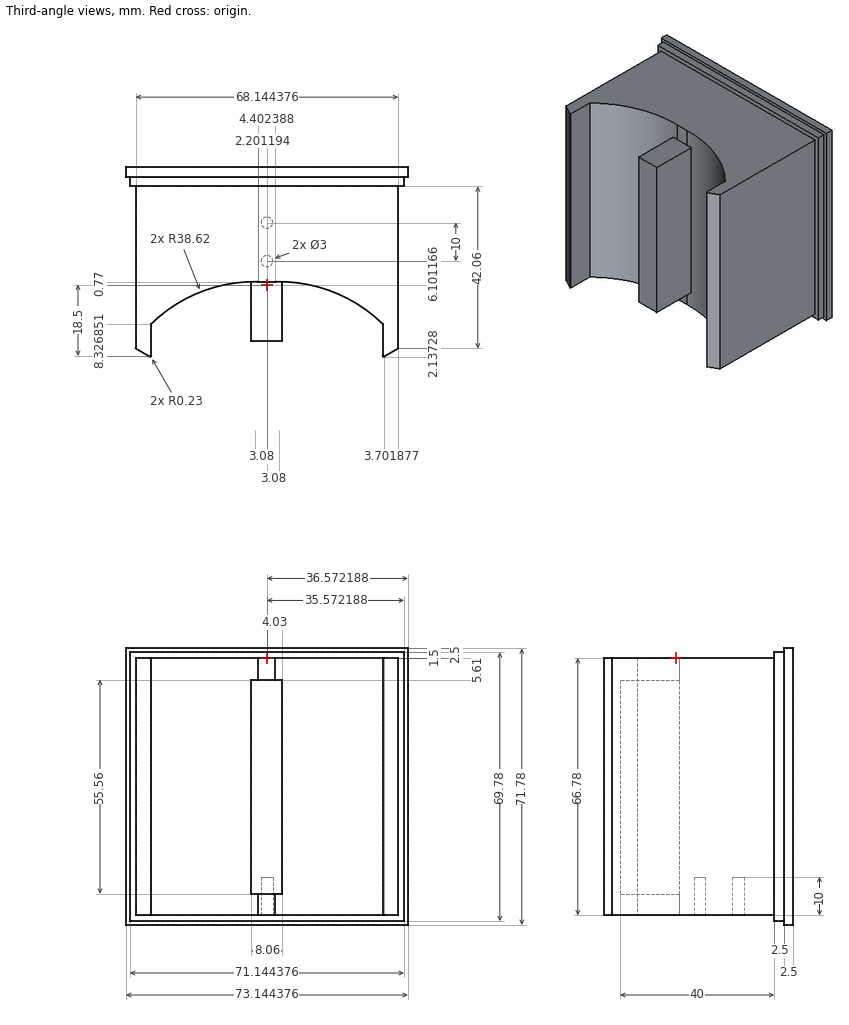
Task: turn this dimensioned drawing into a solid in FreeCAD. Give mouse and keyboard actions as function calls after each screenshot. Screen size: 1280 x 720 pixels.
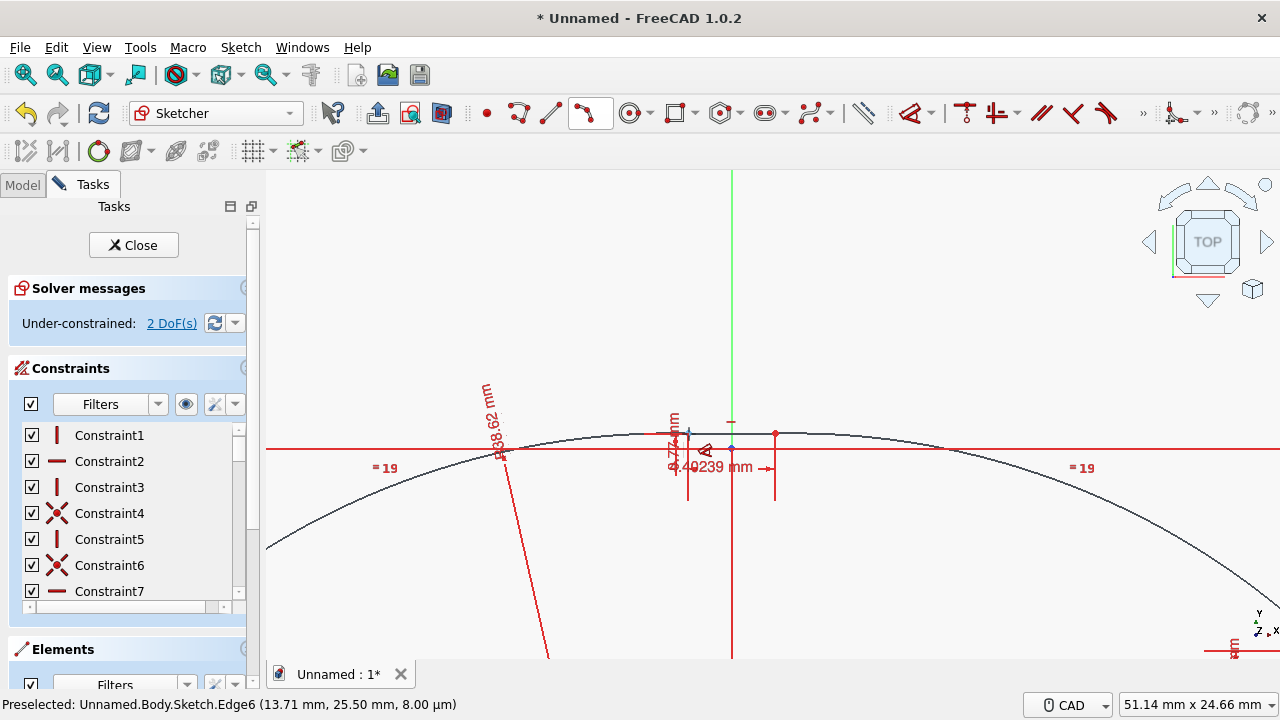
click(688, 434)
click(710, 400)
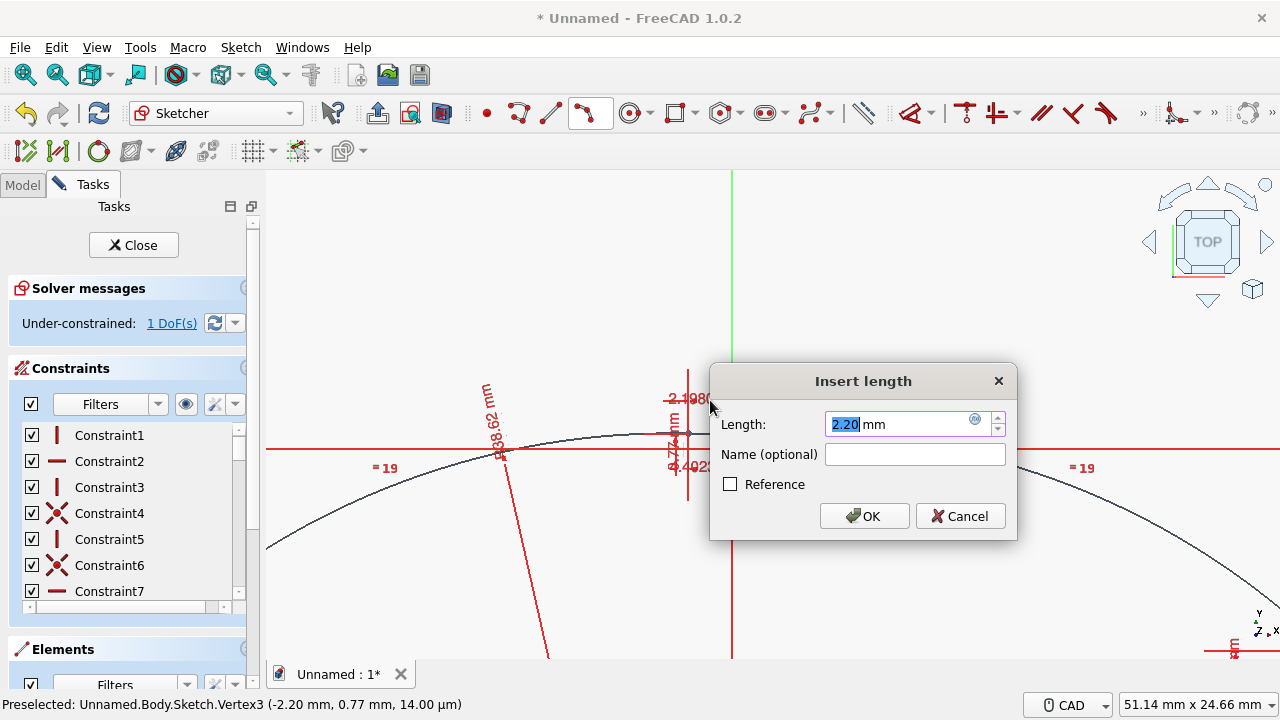
text(2.201194)
key(Return)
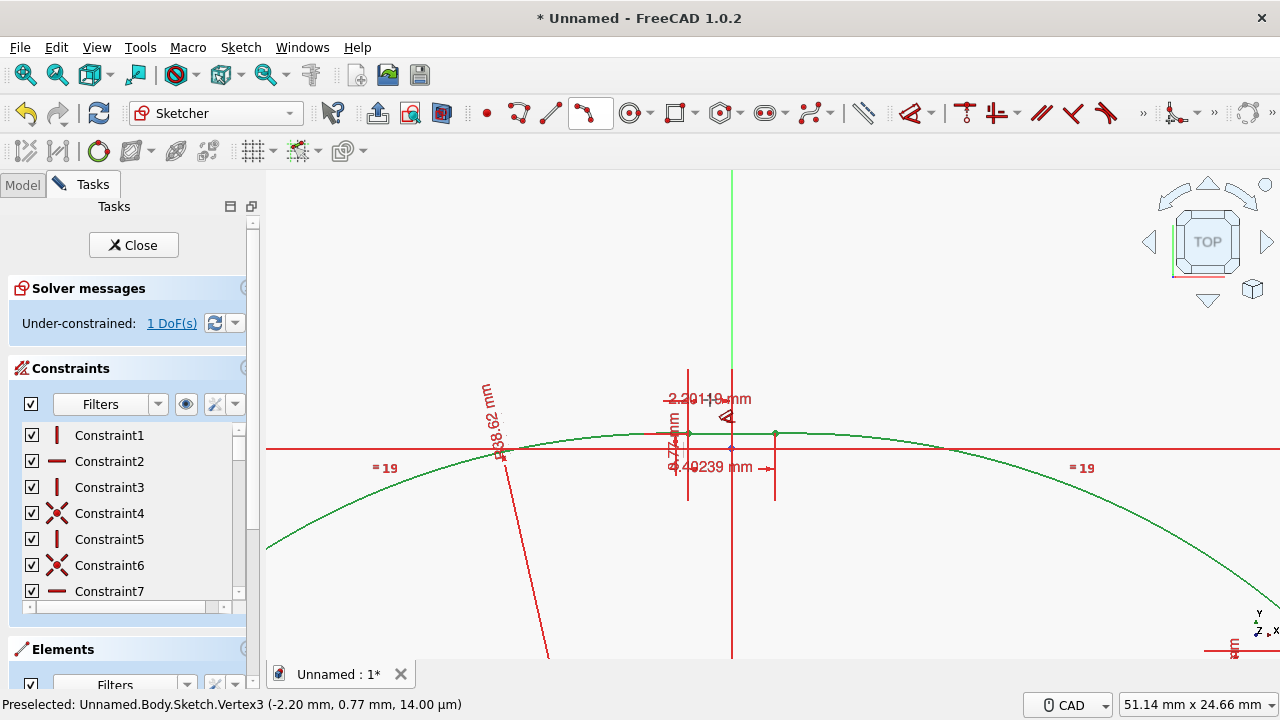
scroll(689, 434, down, 5)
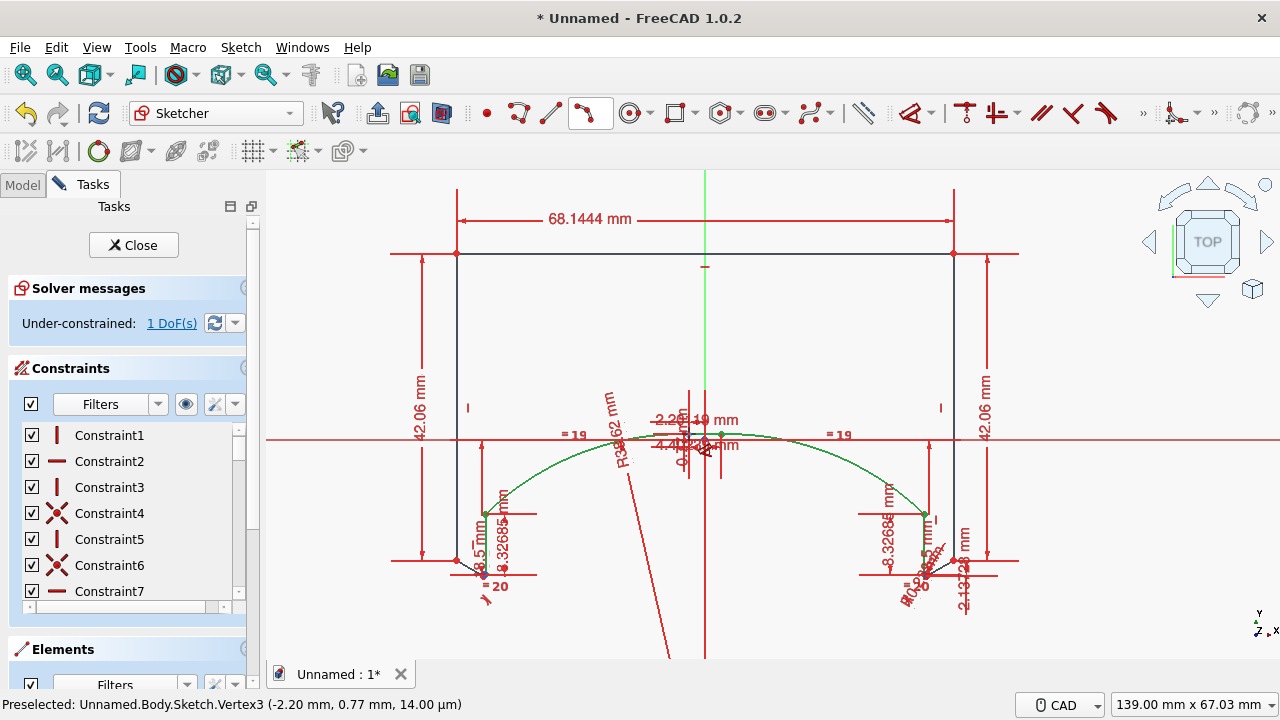
scroll(935, 572, up, 2)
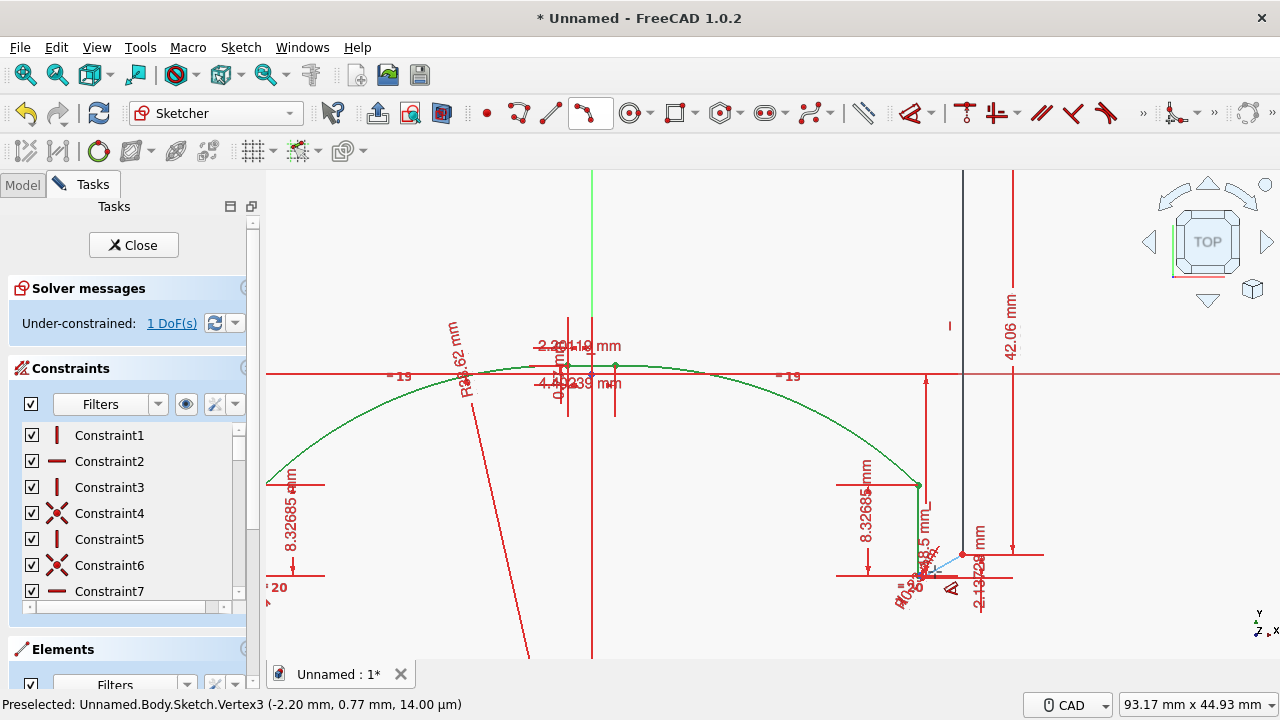
click(934, 571)
click(942, 612)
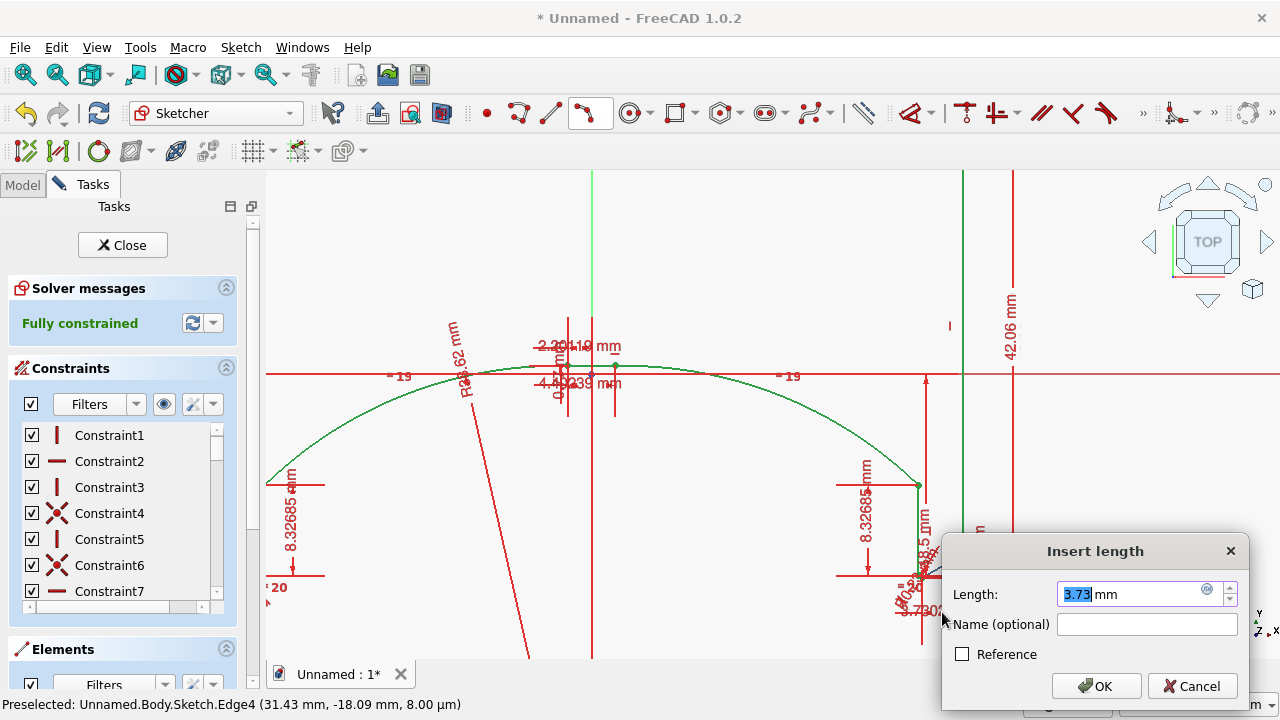
text(3.701877)
key(Return)
key(Escape)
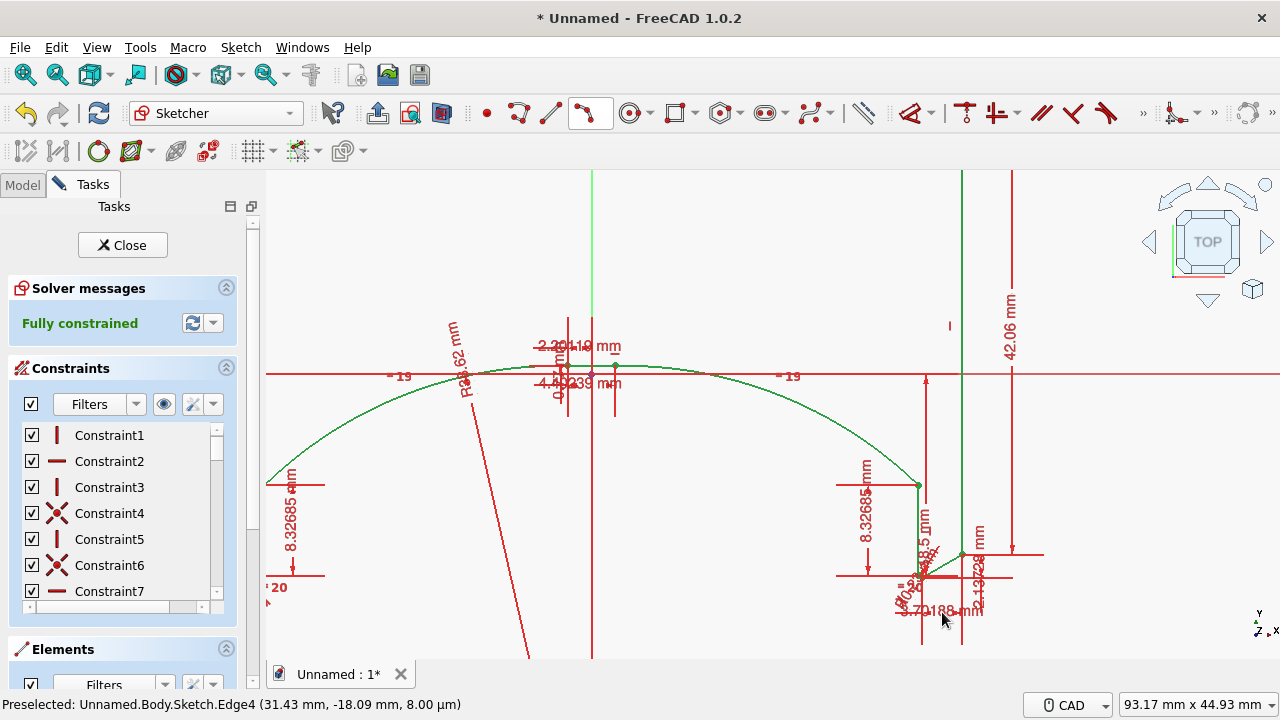
click(123, 245)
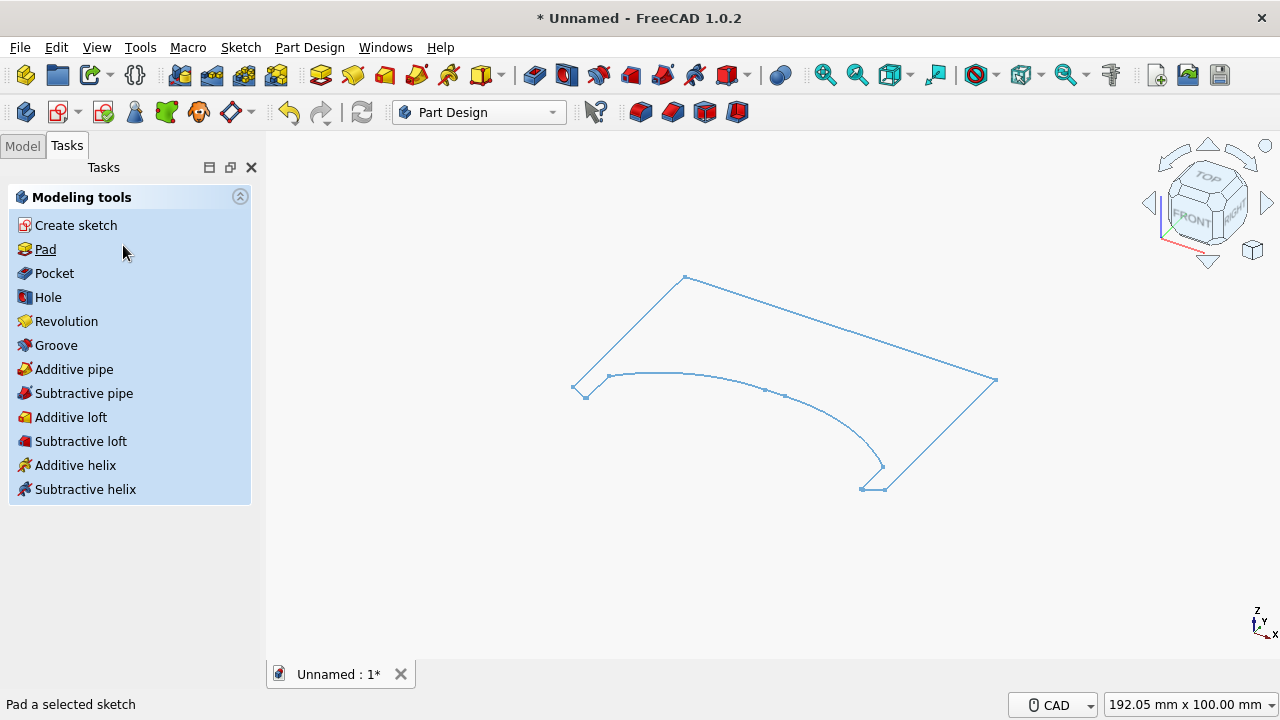
click(322, 76)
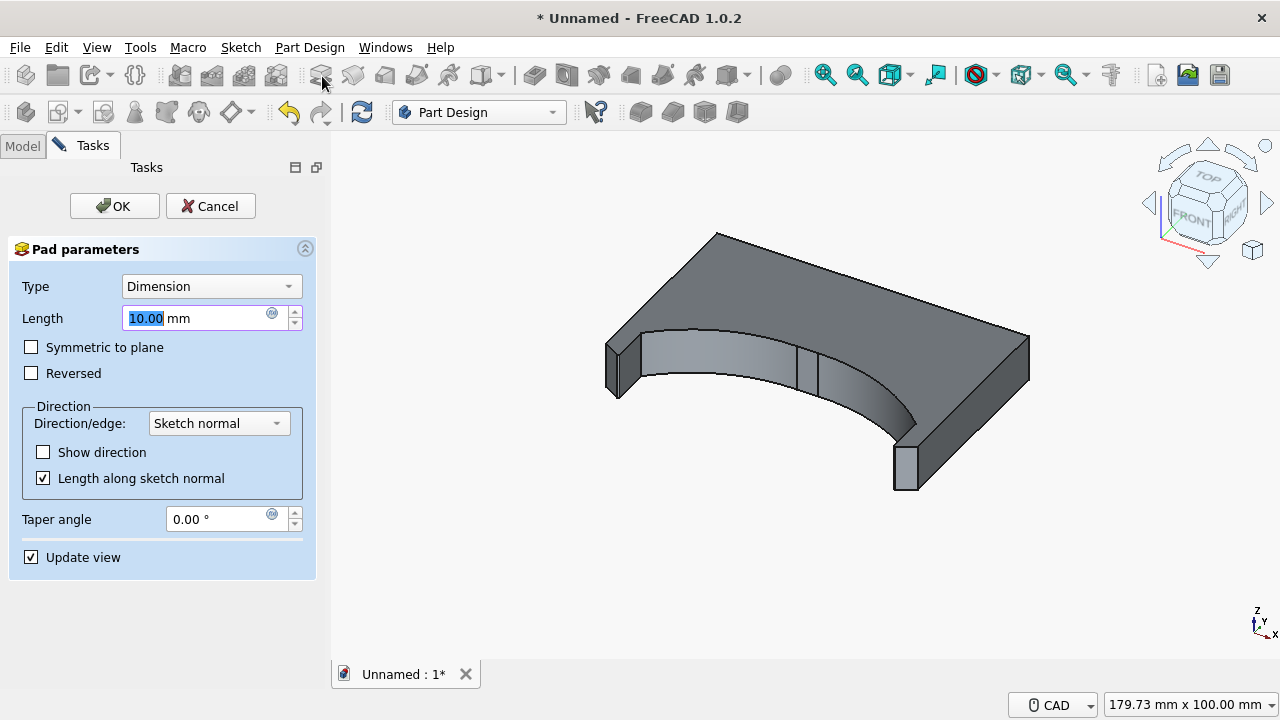
text(66.78)
key(Tab)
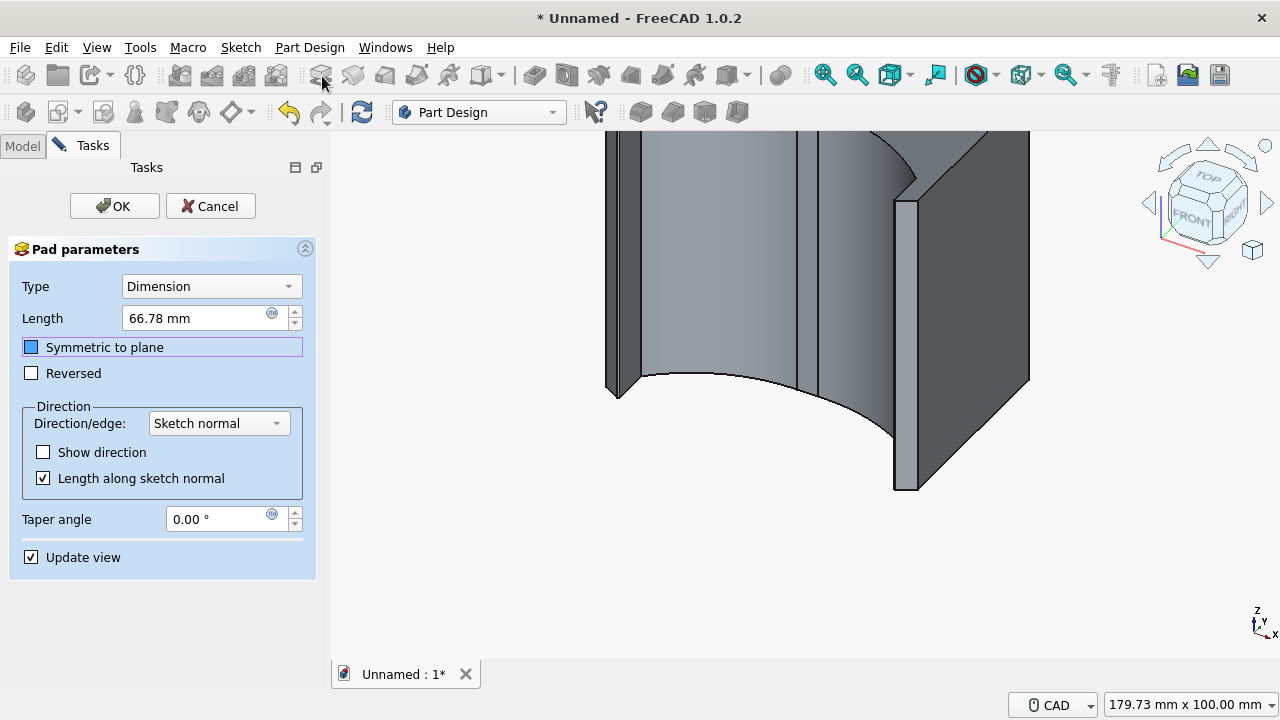
click(30, 373)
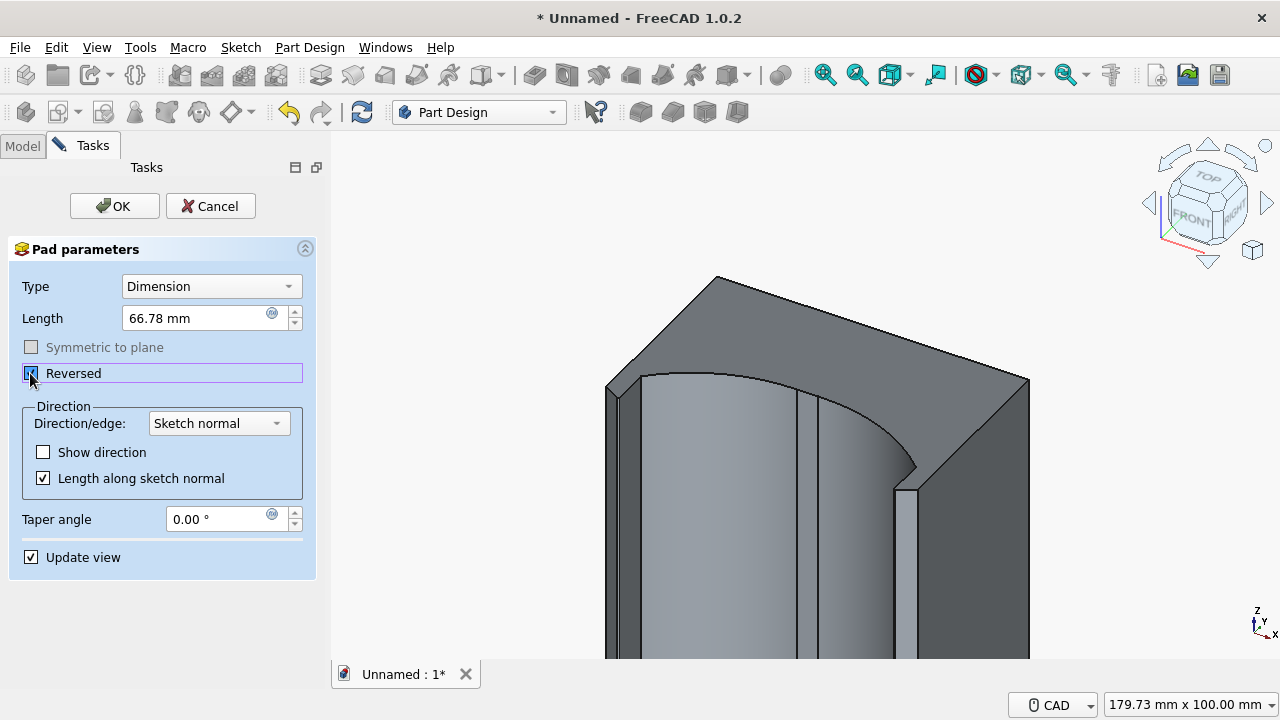
click(115, 206)